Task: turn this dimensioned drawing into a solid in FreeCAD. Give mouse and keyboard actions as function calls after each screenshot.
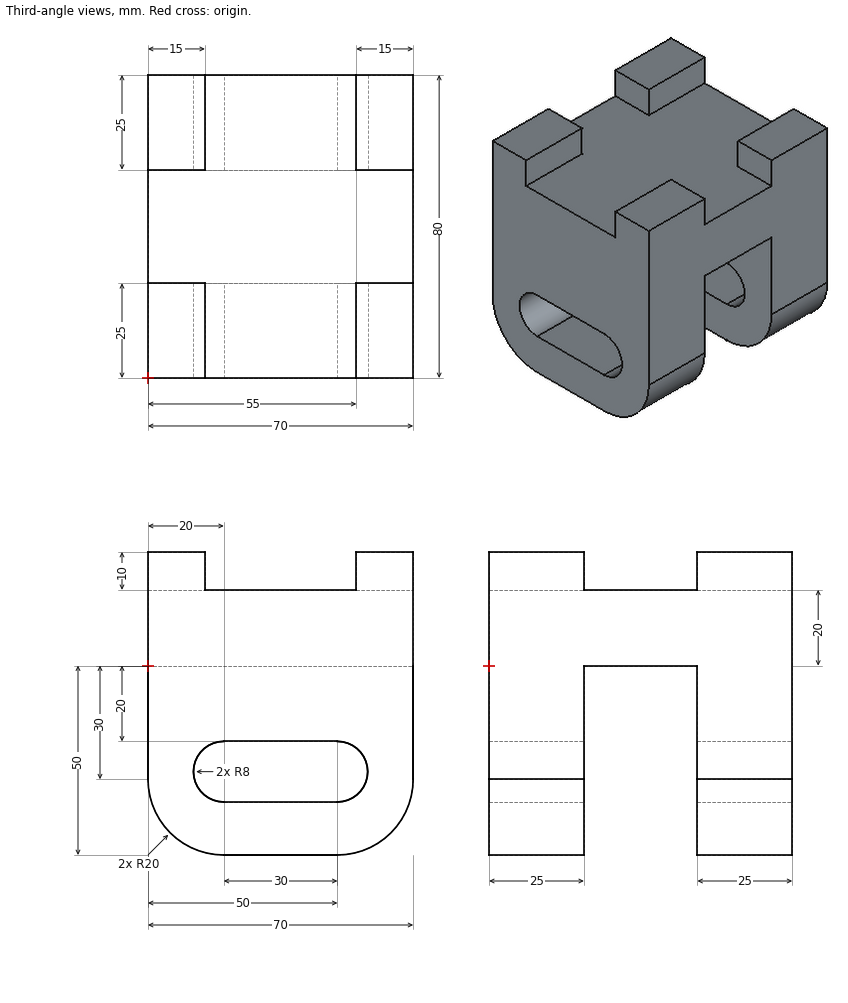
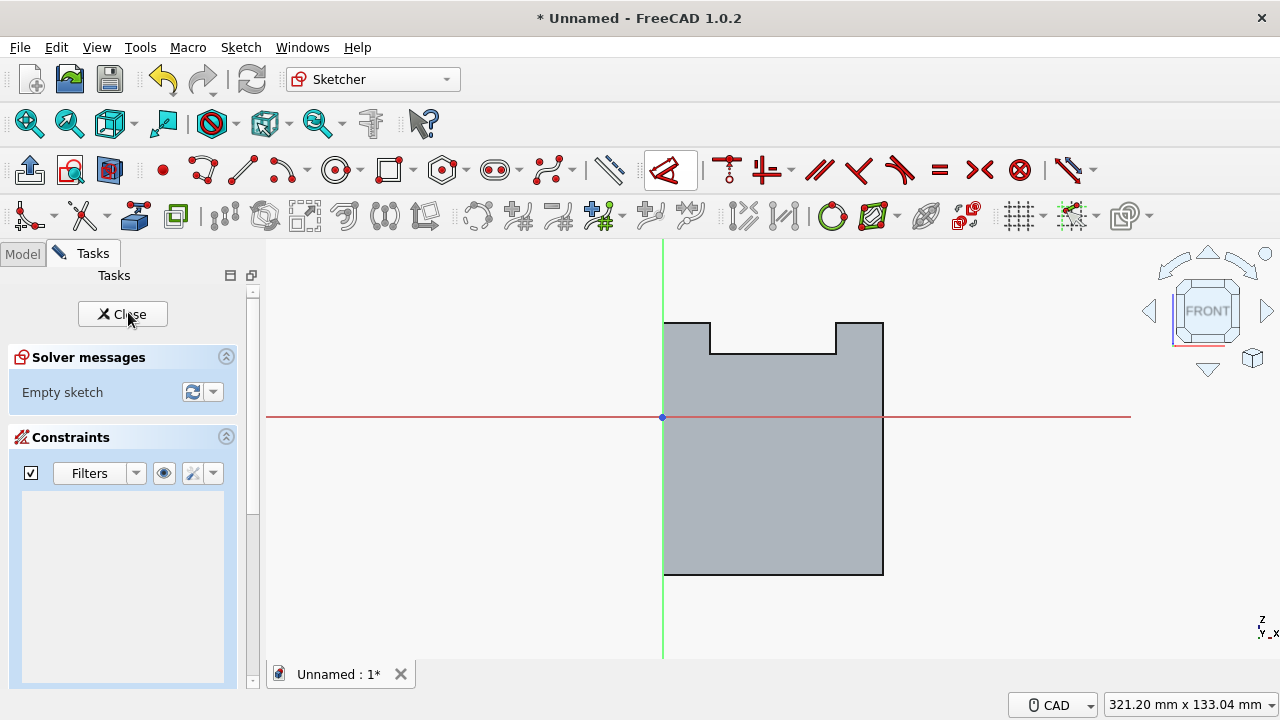
scroll(912, 593, up, 2)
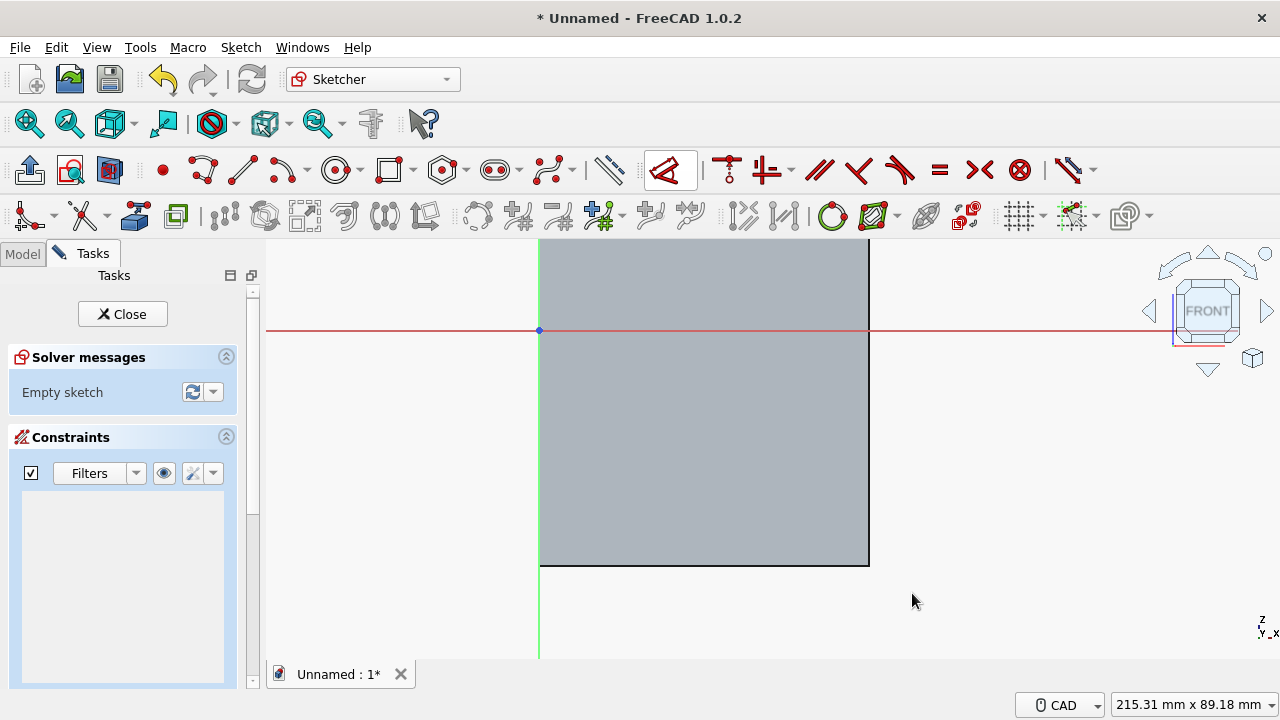
key(g)
key(r)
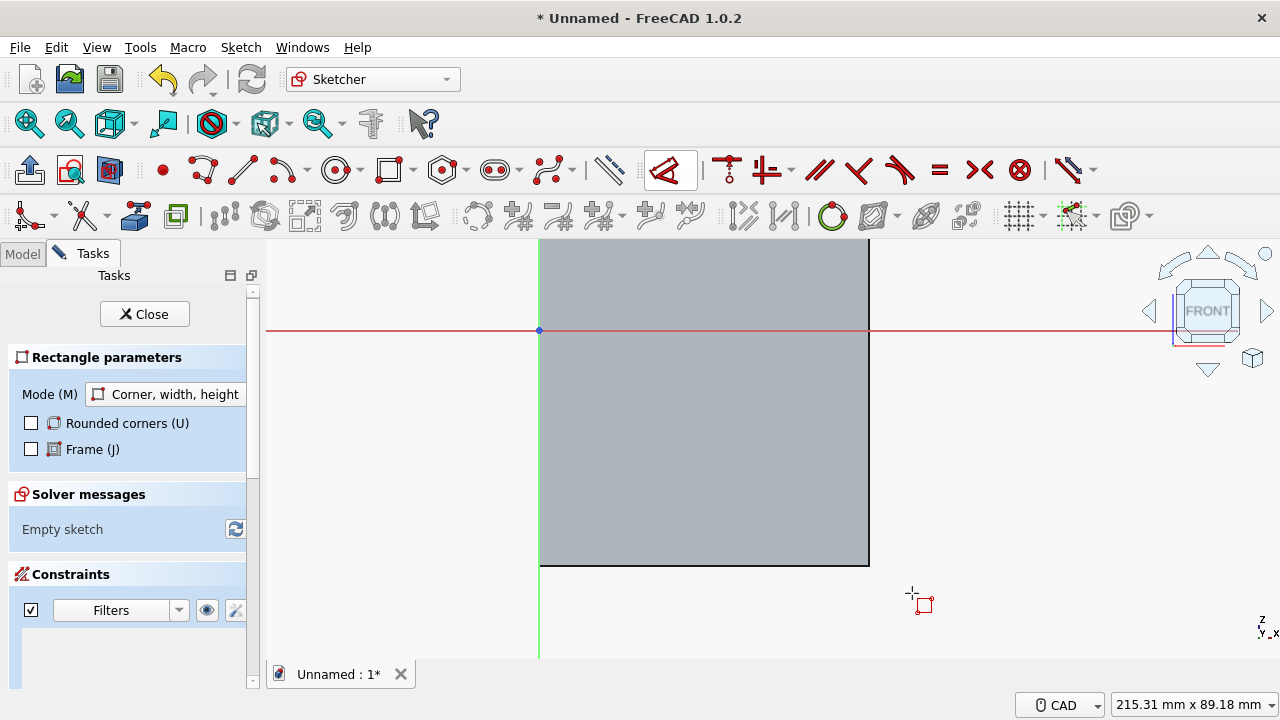
click(539, 331)
move(869, 566)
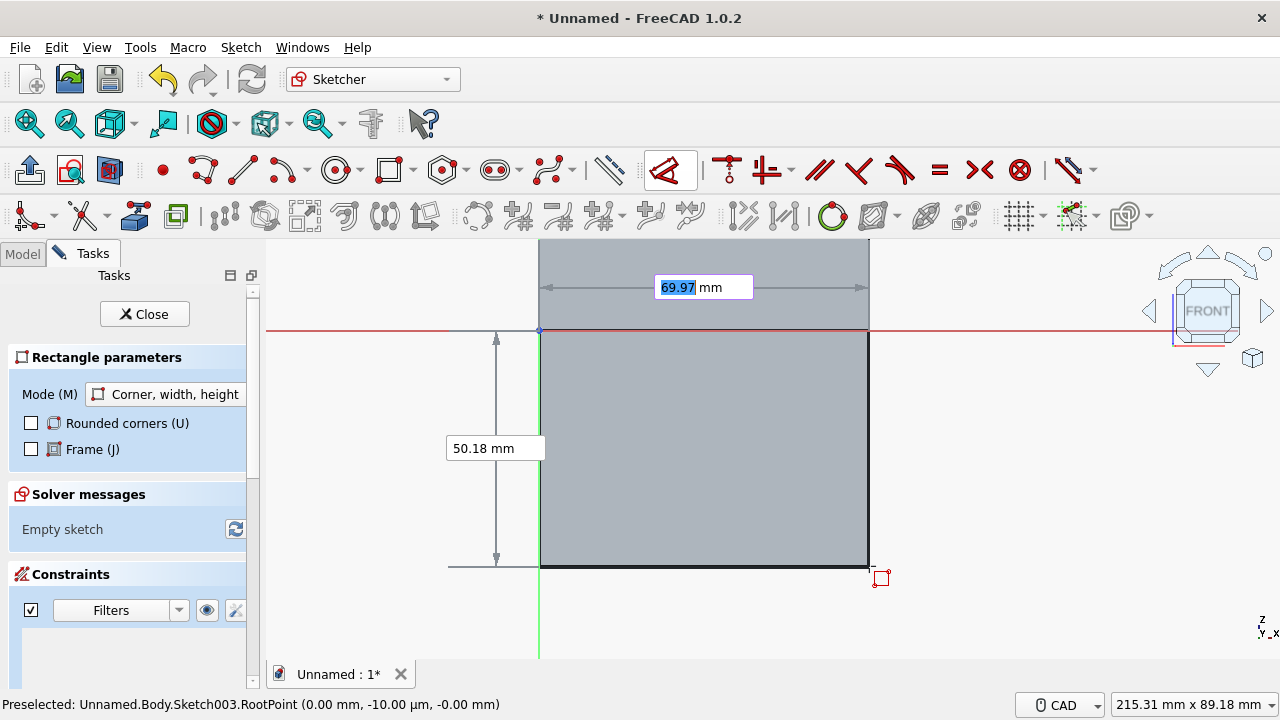
text(70)
key(Tab)
text(50)
key(Return)
key(Escape)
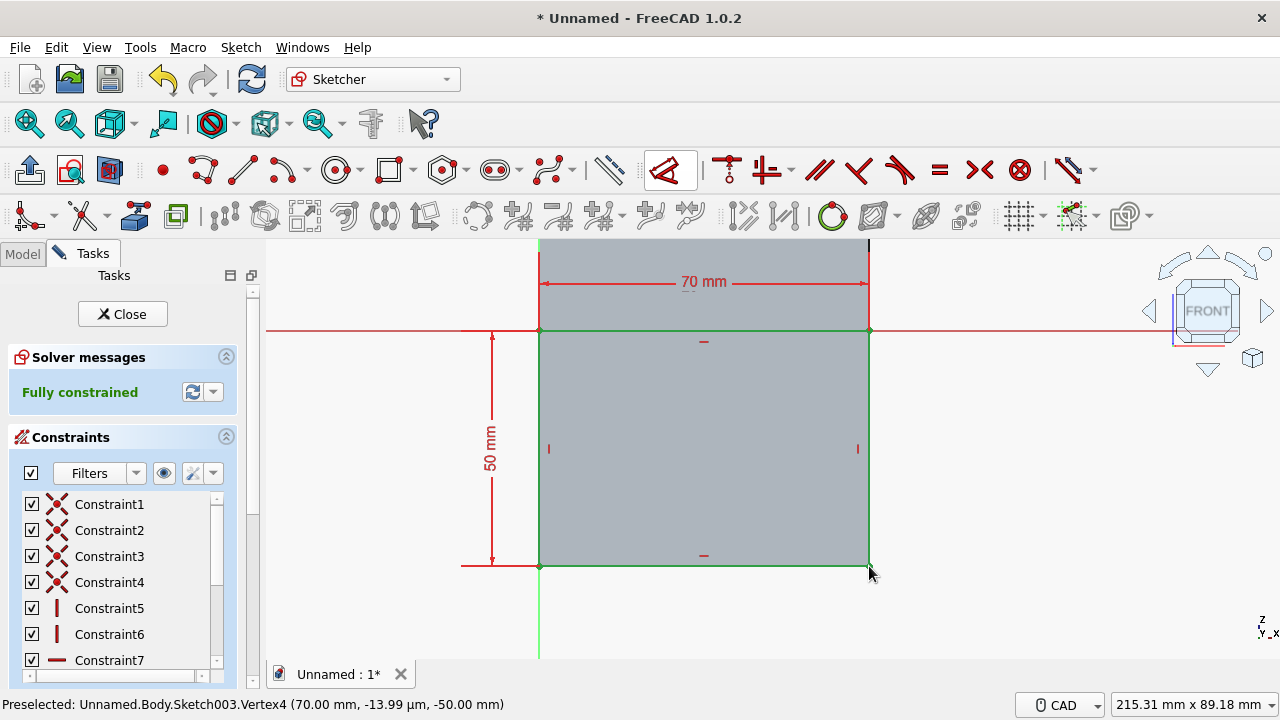
click(123, 314)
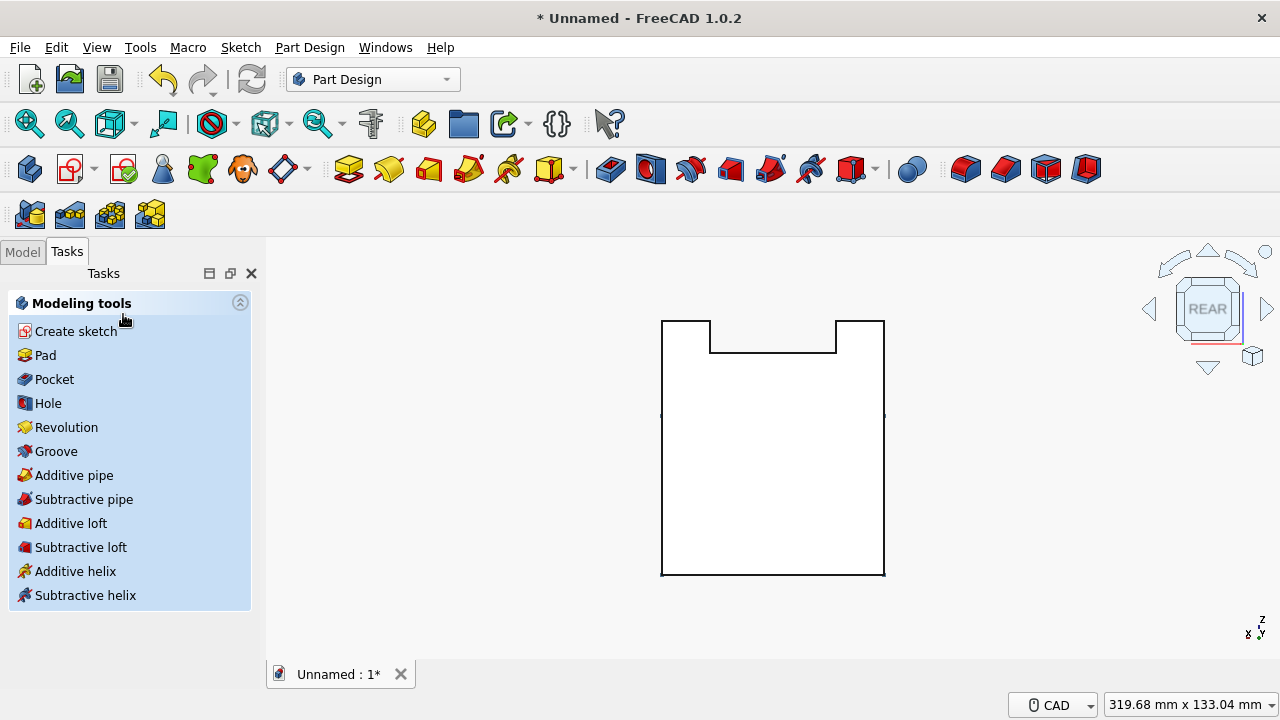
click(350, 170)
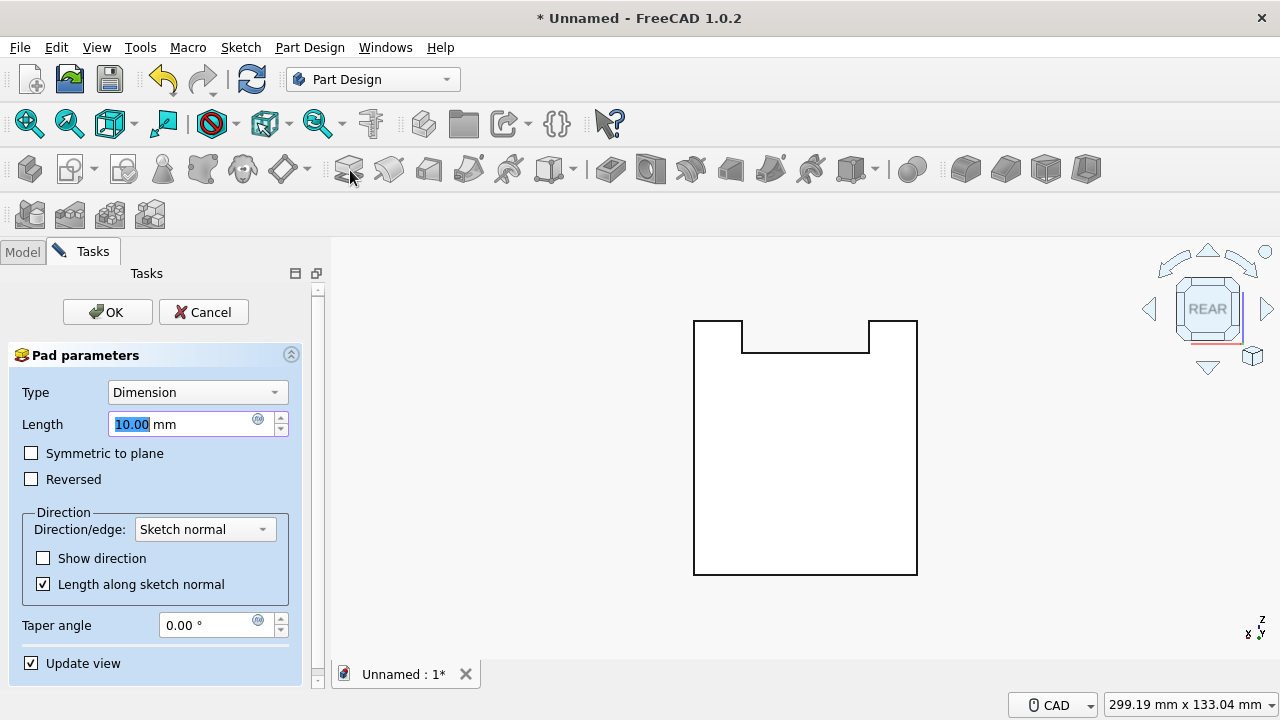
text(25)
key(Tab)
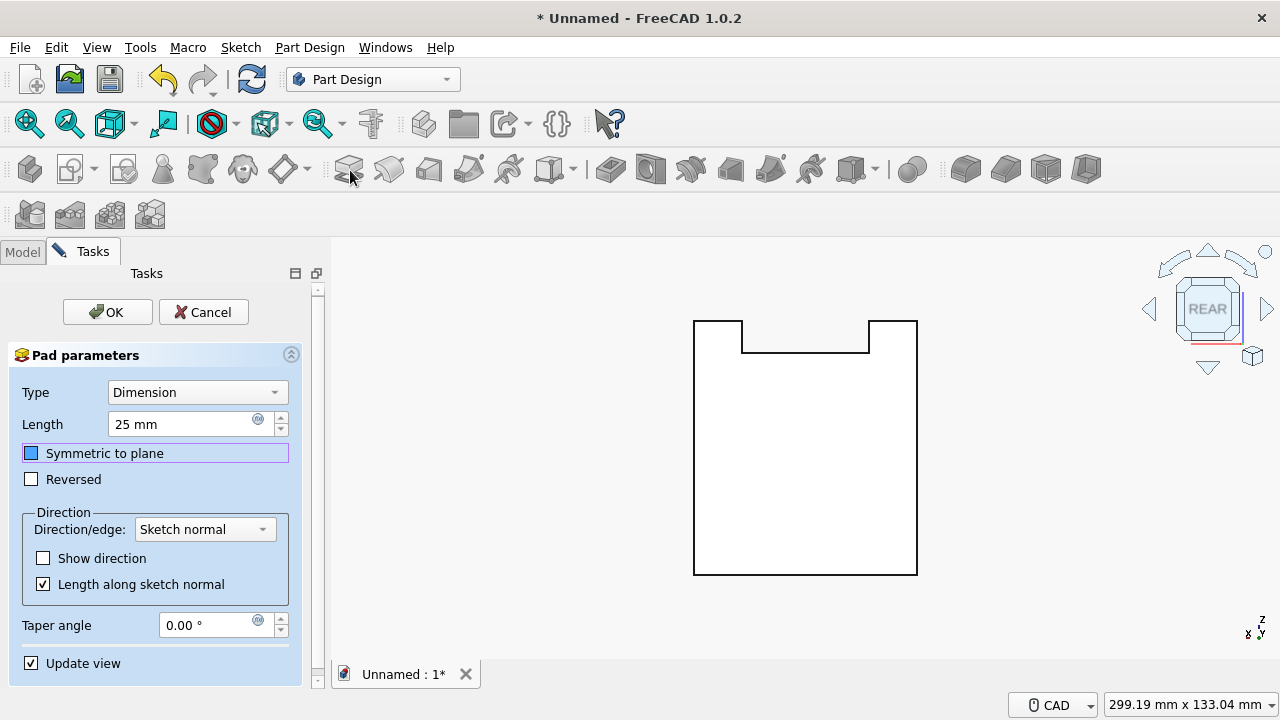
click(30, 479)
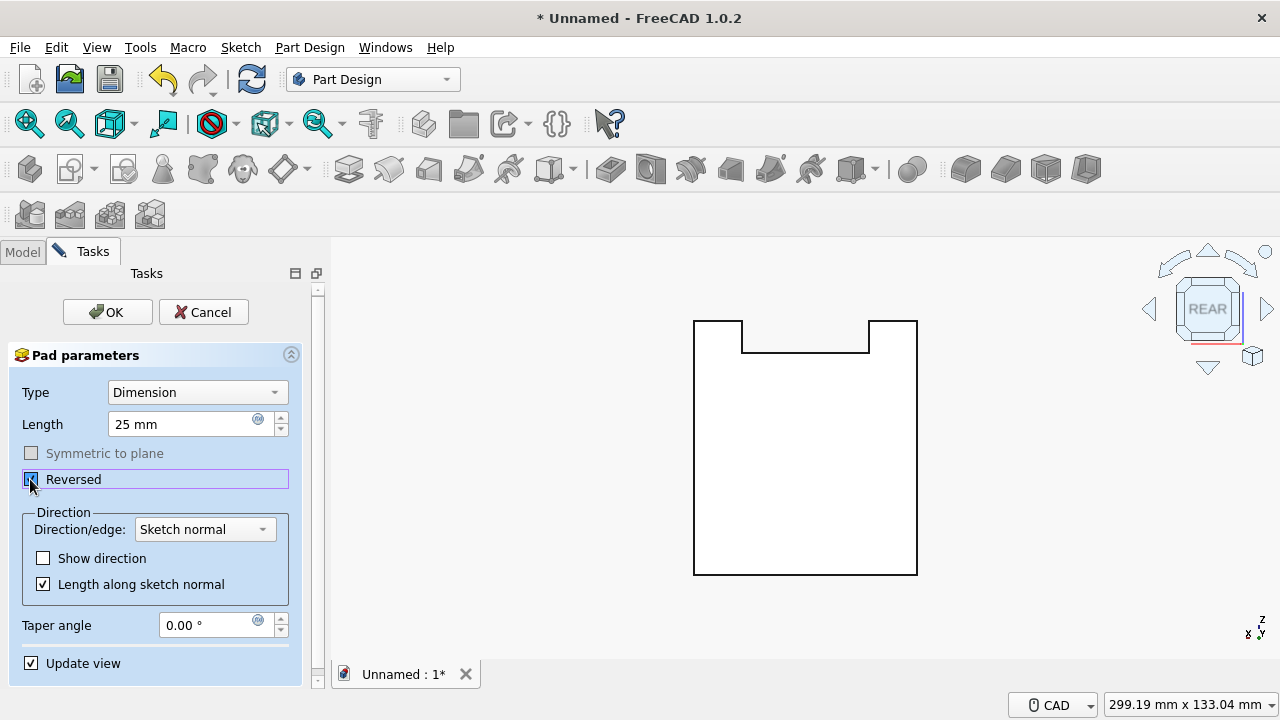
click(108, 312)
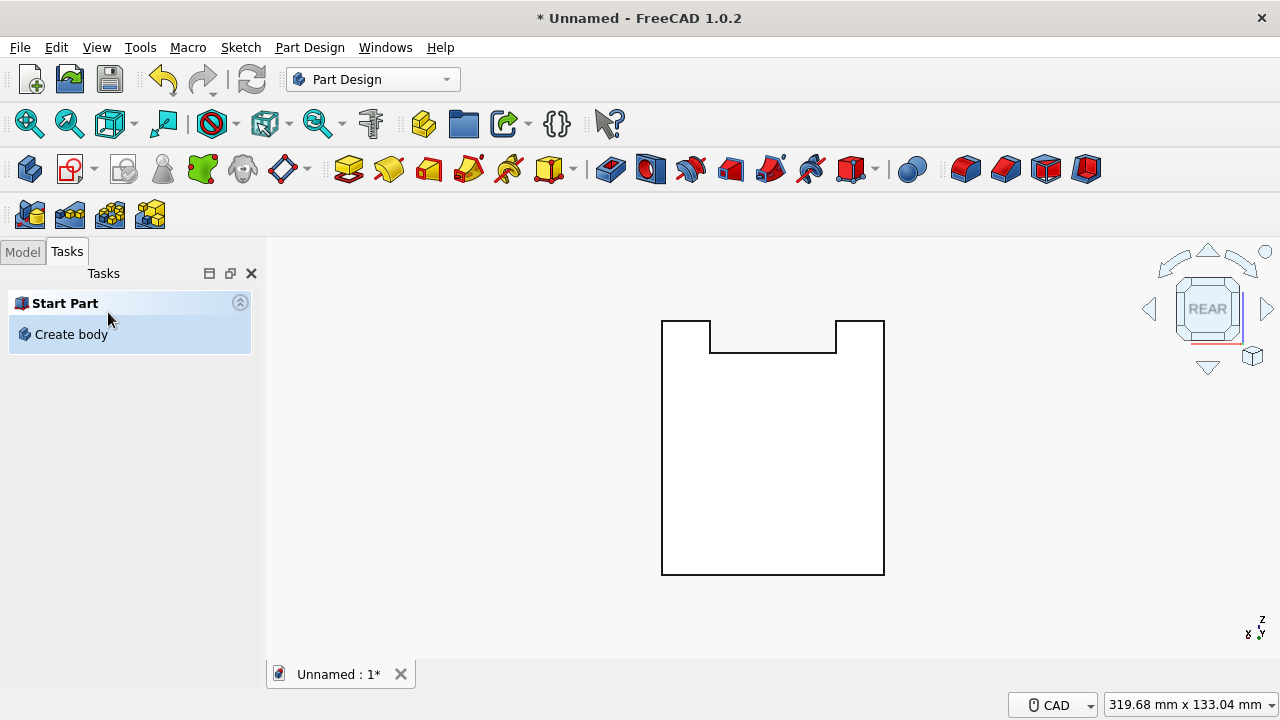
key(0)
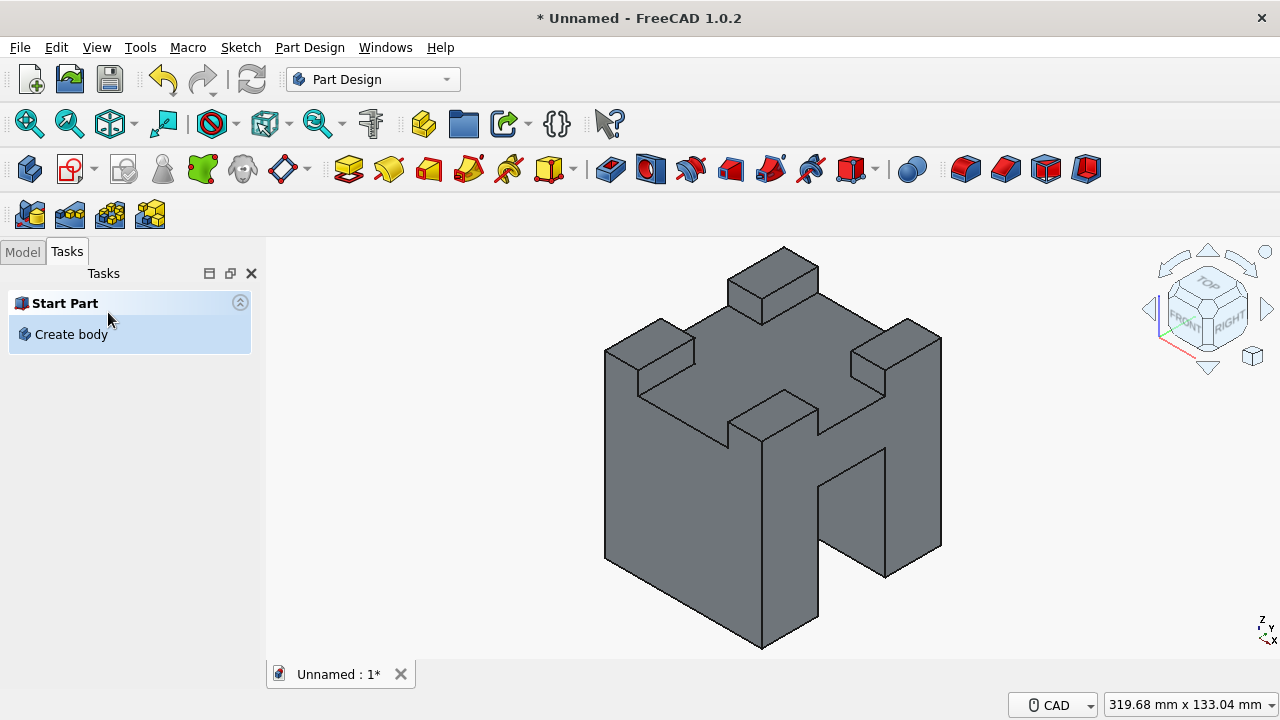
click(683, 499)